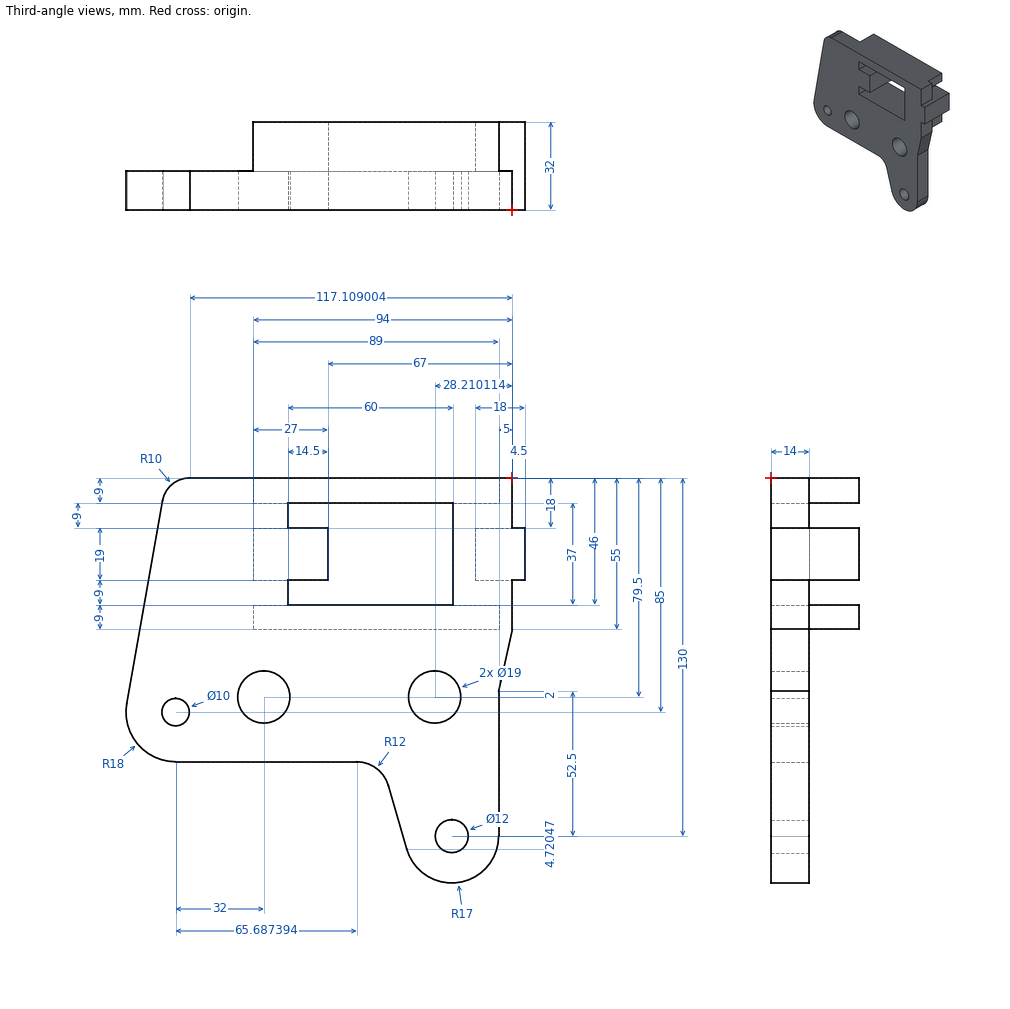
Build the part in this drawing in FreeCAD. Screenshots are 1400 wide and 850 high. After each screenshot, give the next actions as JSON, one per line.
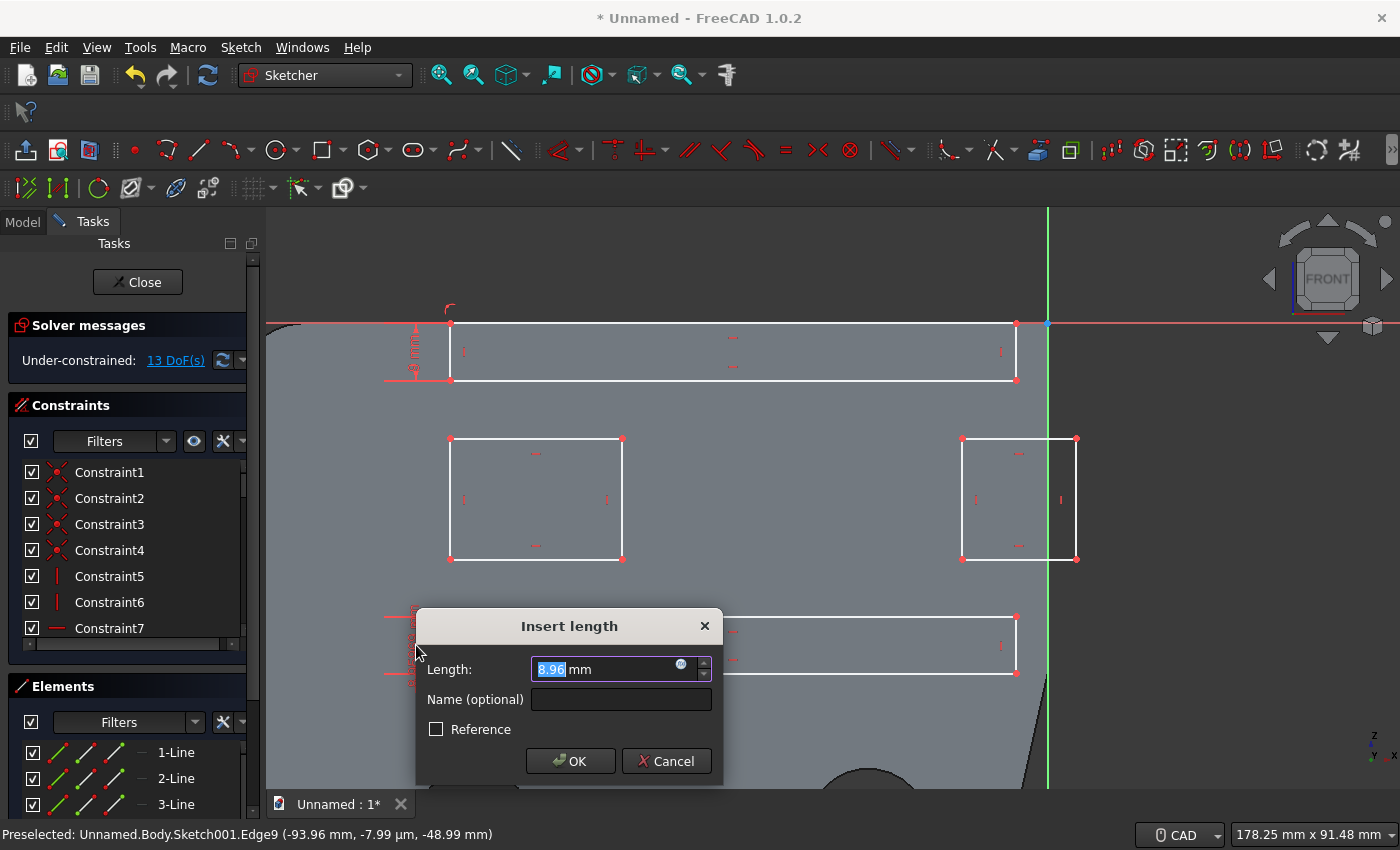
{"action": "type", "text": "9"}
{"action": "key", "text": "Return"}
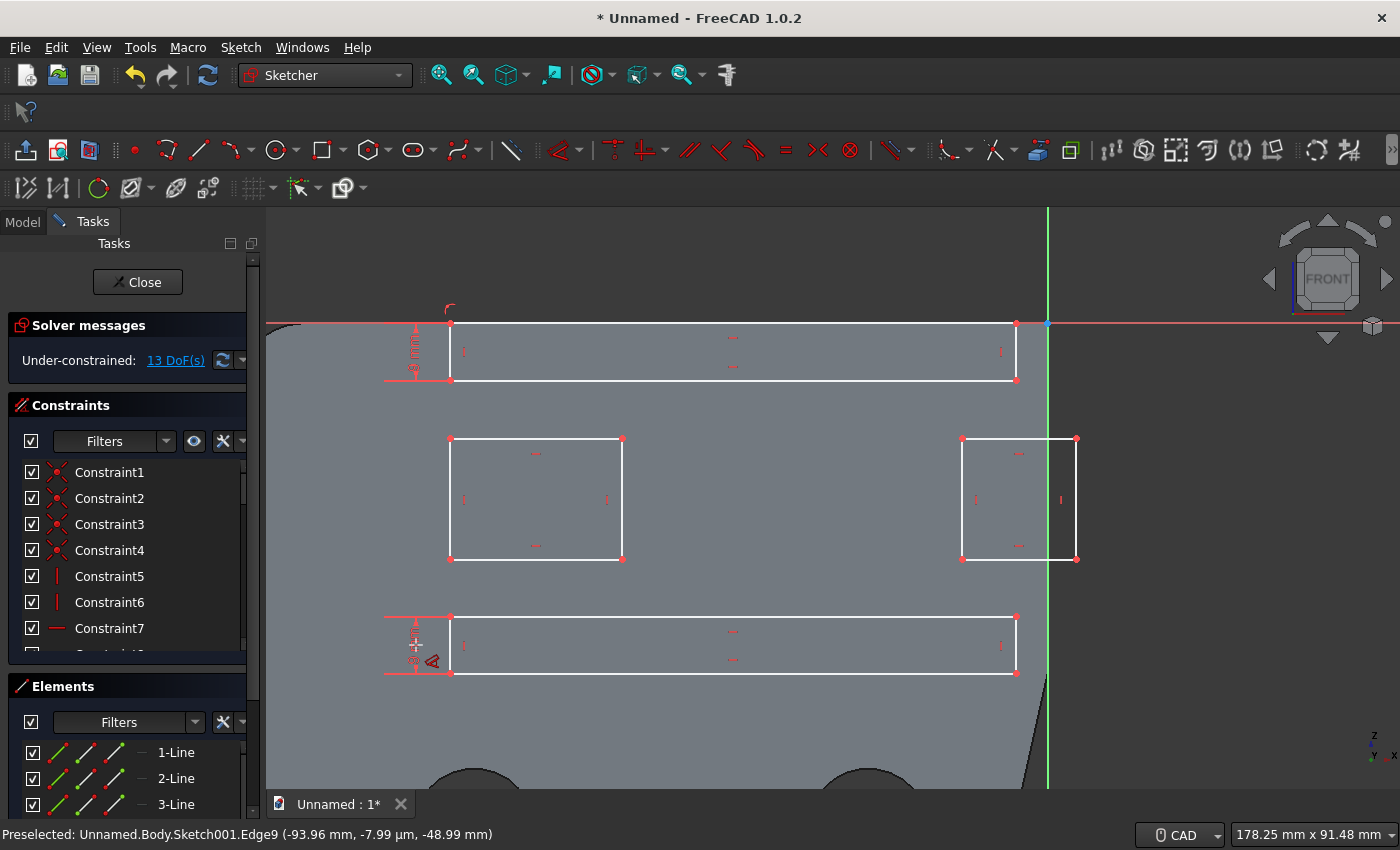
{"action": "left_click", "coordinate": [620, 381]}
{"action": "left_click", "coordinate": [733, 347]}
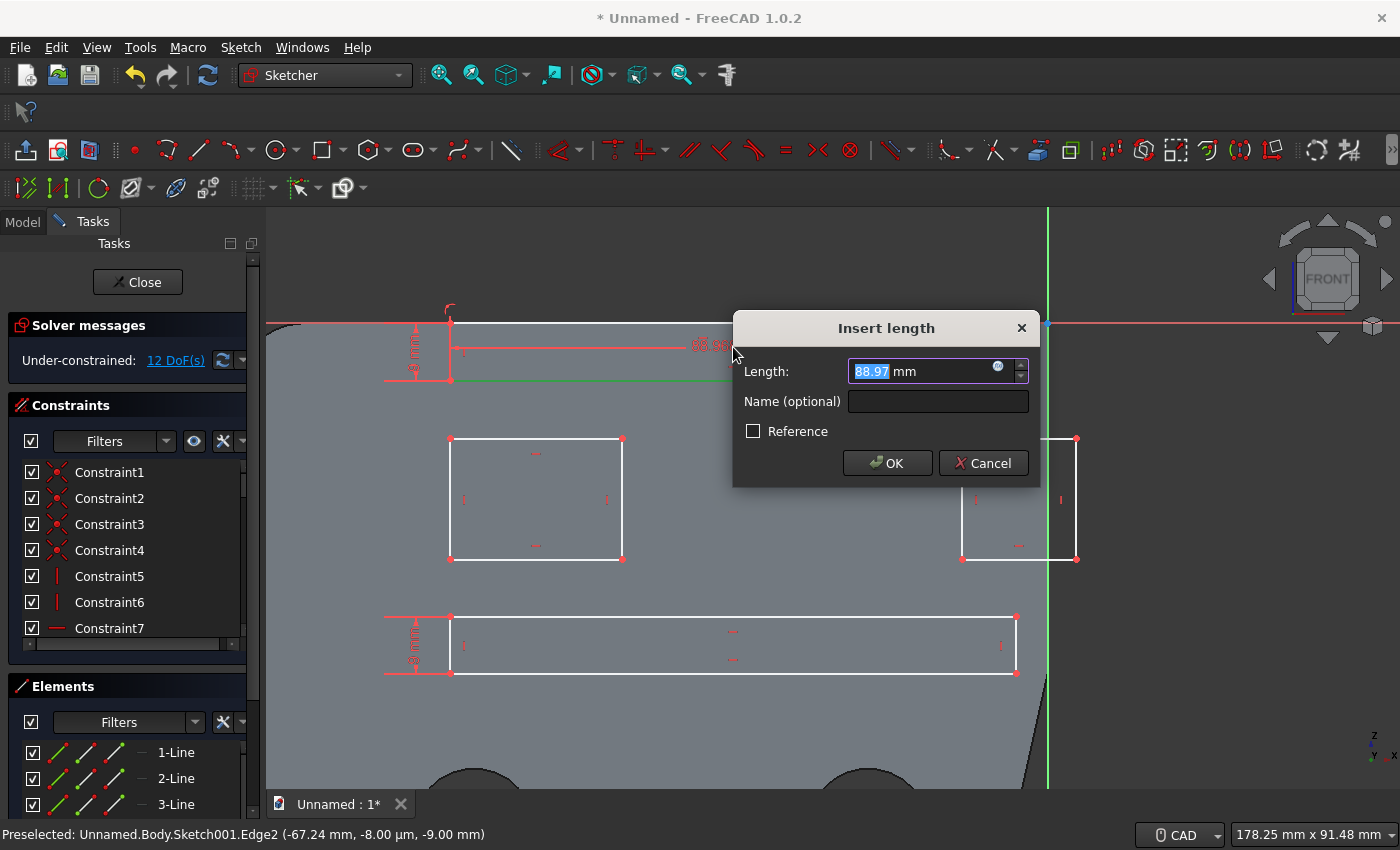
{"action": "type", "text": "89"}
{"action": "key", "text": "Return"}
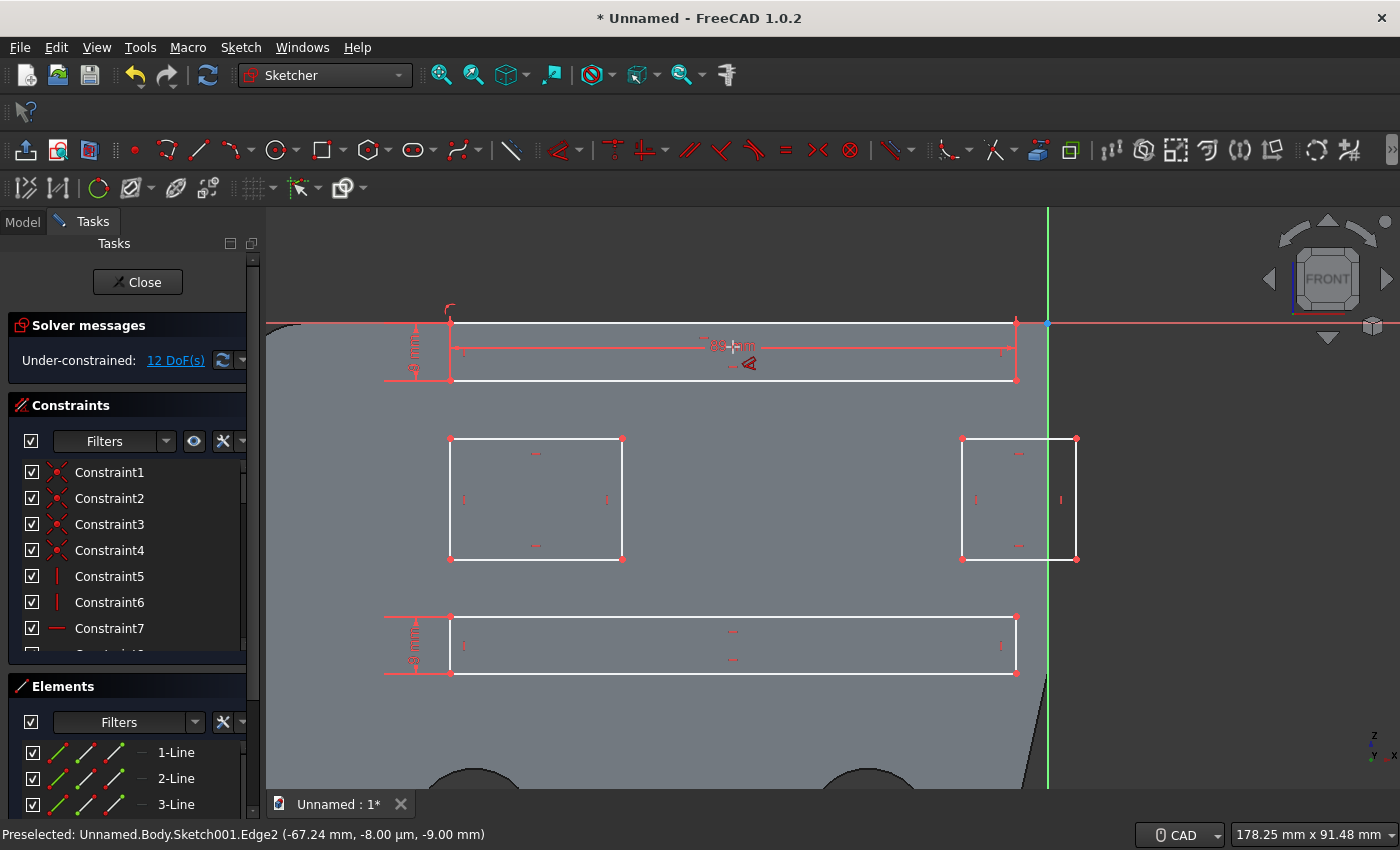
{"action": "left_click", "coordinate": [450, 475]}
{"action": "left_click", "coordinate": [416, 500]}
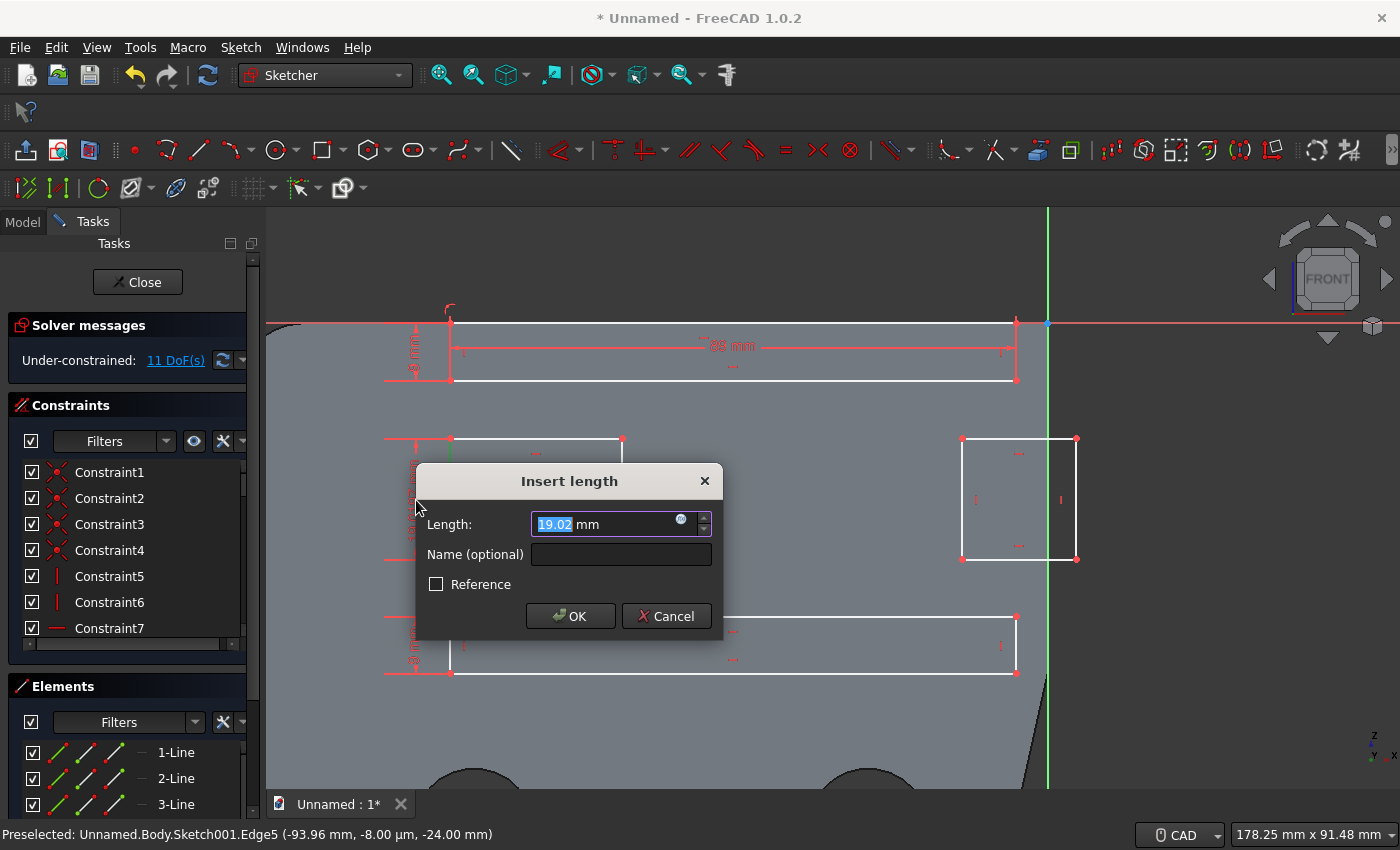
{"action": "type", "text": "19"}
{"action": "key", "text": "Return"}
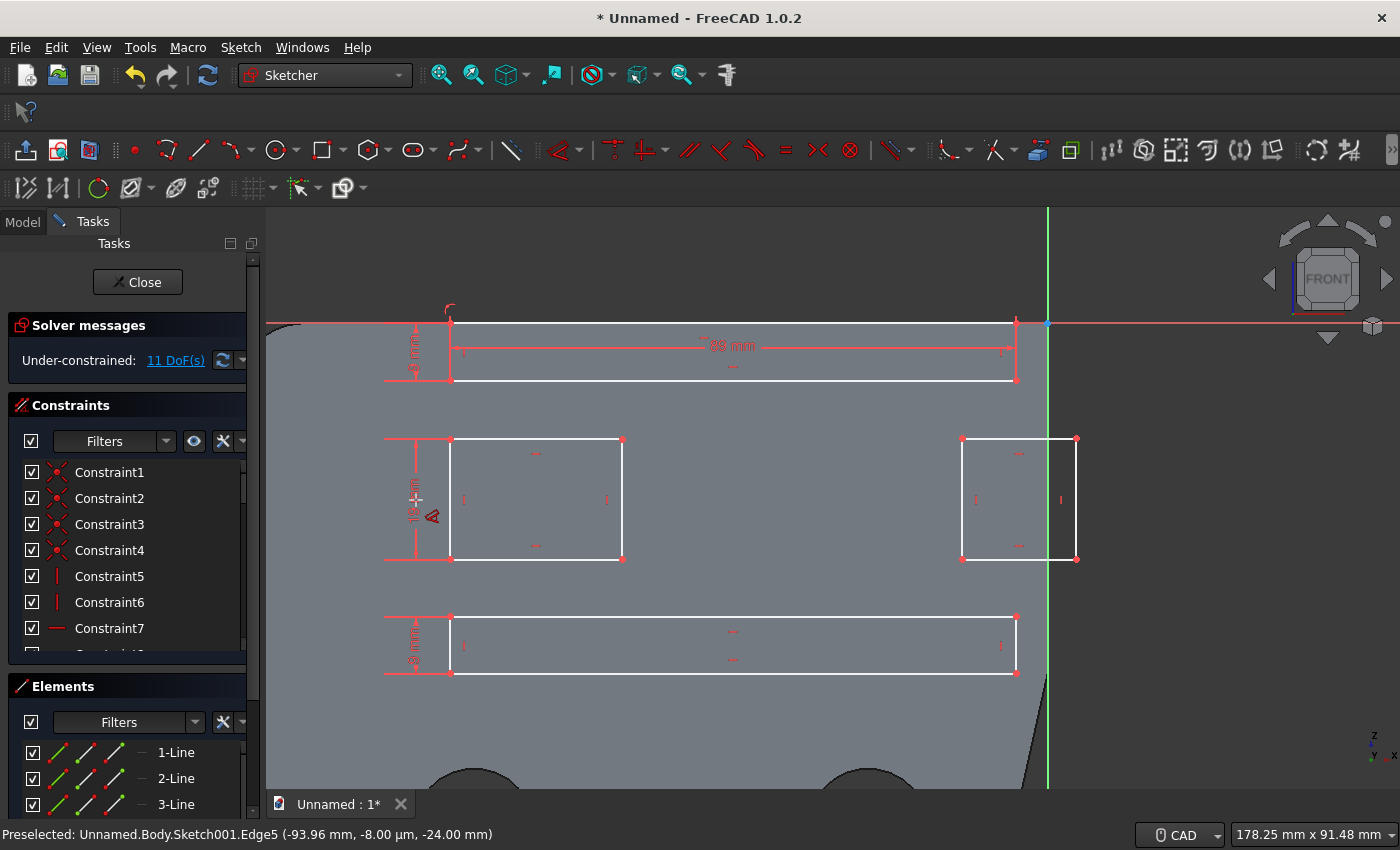
{"action": "left_click", "coordinate": [502, 560]}
{"action": "left_click", "coordinate": [536, 594]}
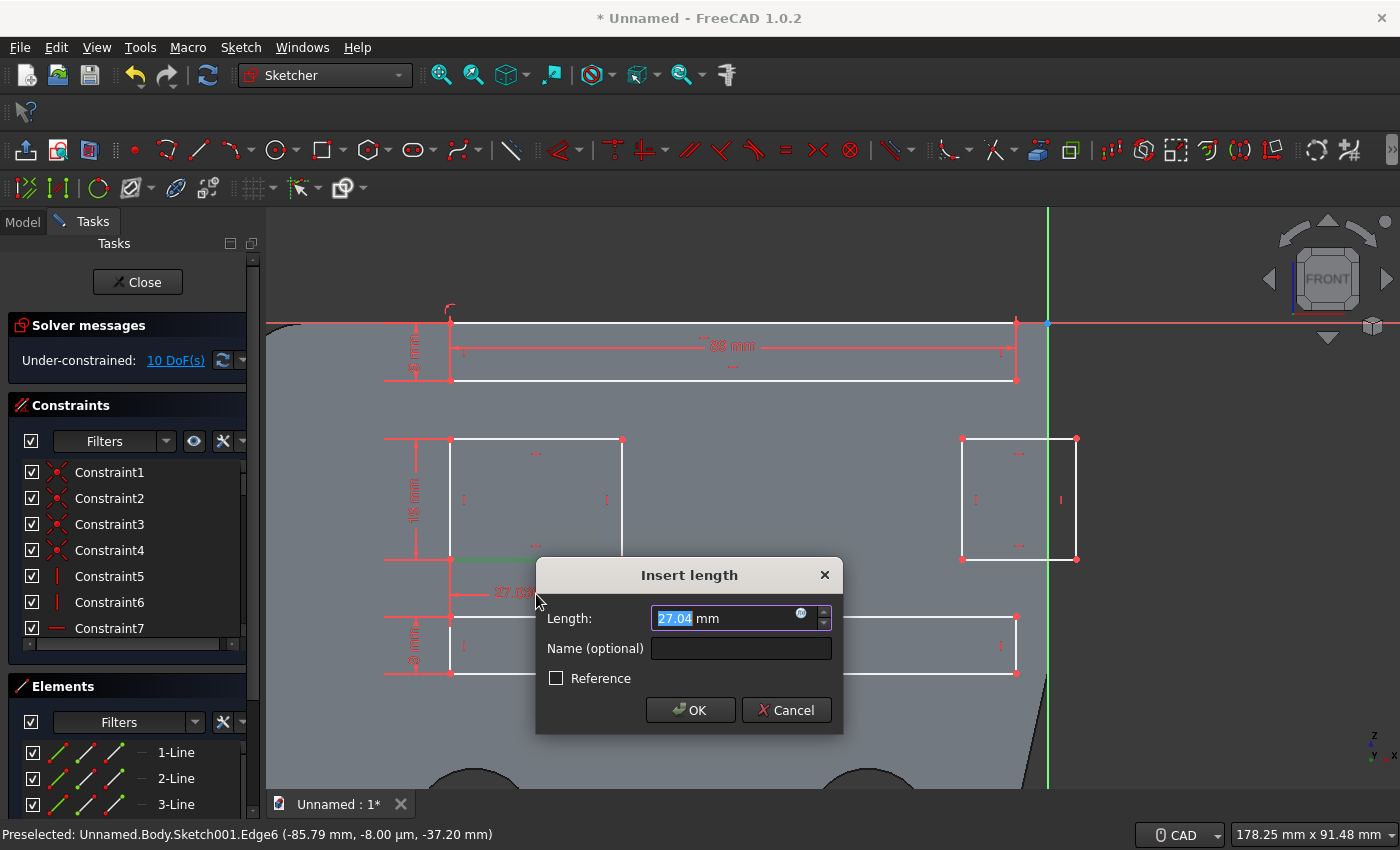
{"action": "type", "text": "27"}
{"action": "key", "text": "Return"}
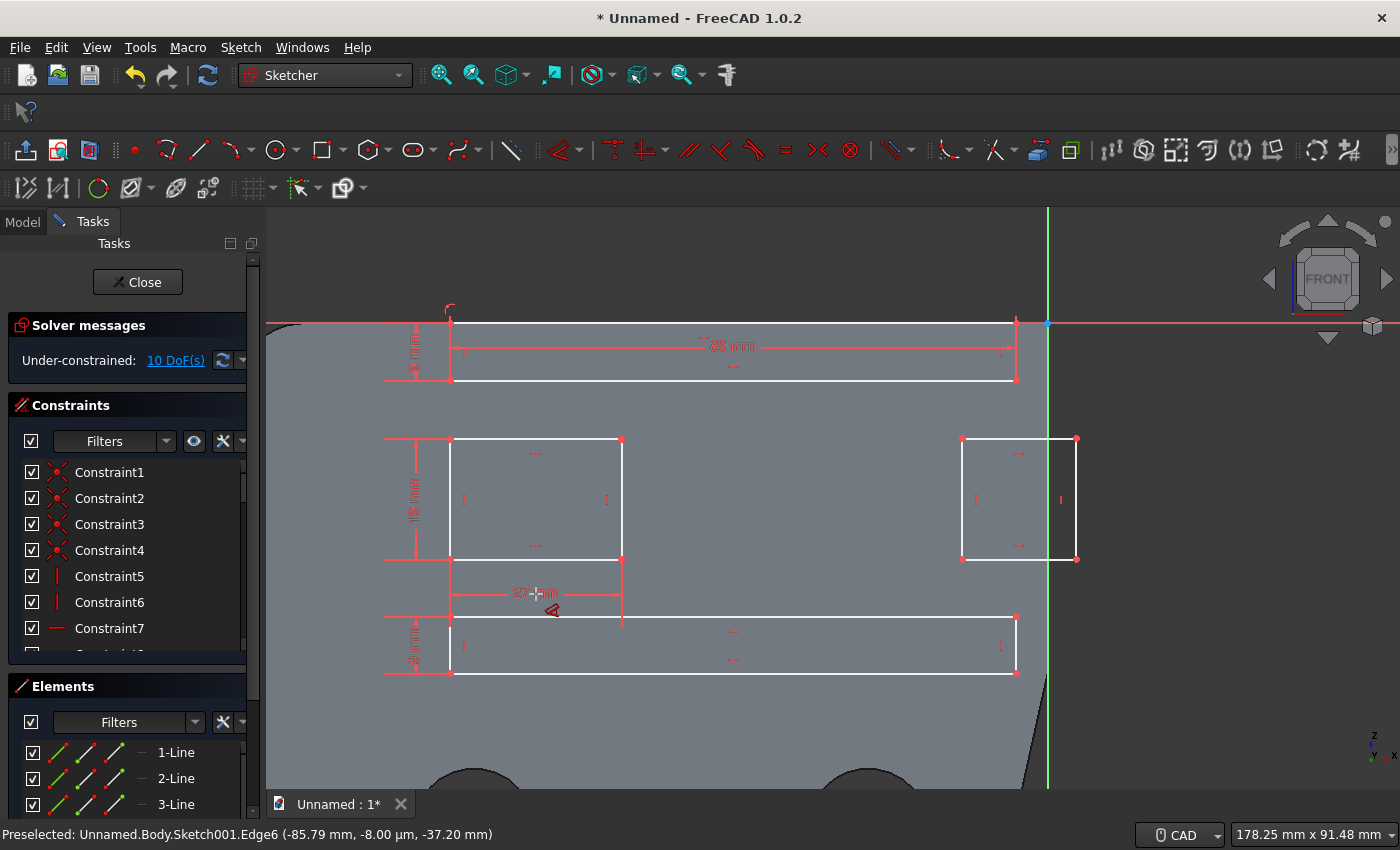
{"action": "left_click", "coordinate": [620, 674]}
{"action": "left_click", "coordinate": [733, 708]}